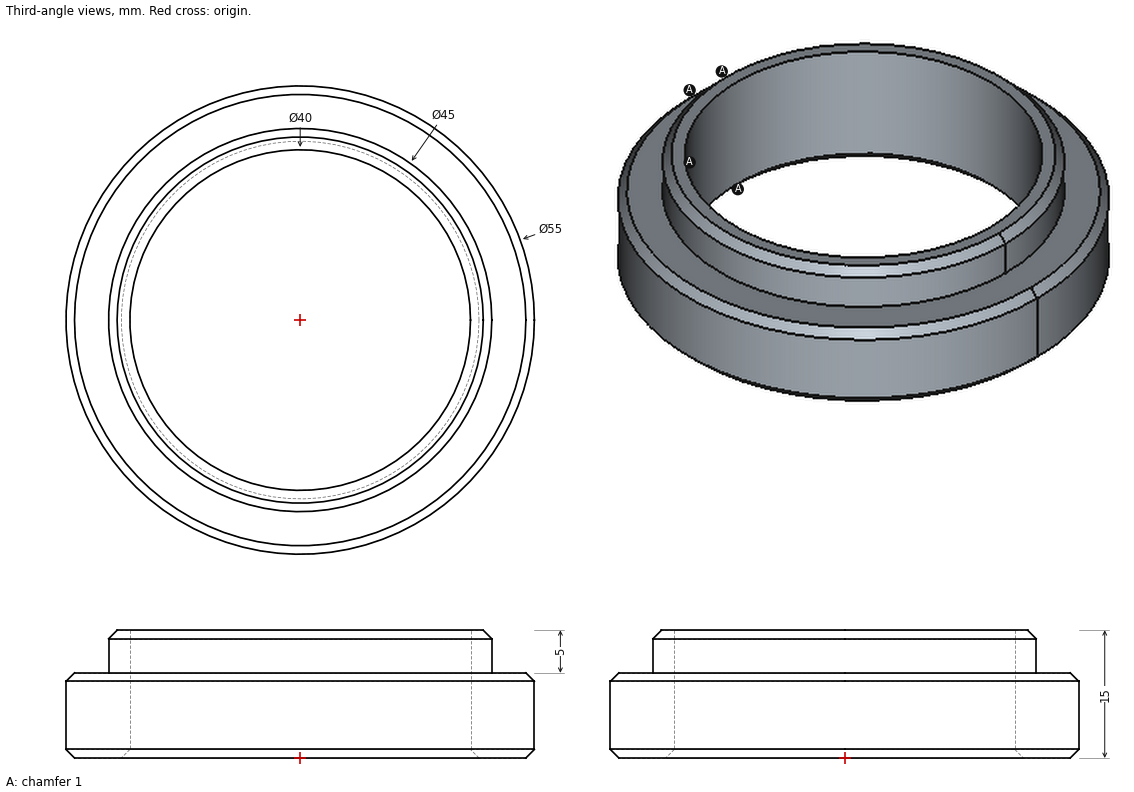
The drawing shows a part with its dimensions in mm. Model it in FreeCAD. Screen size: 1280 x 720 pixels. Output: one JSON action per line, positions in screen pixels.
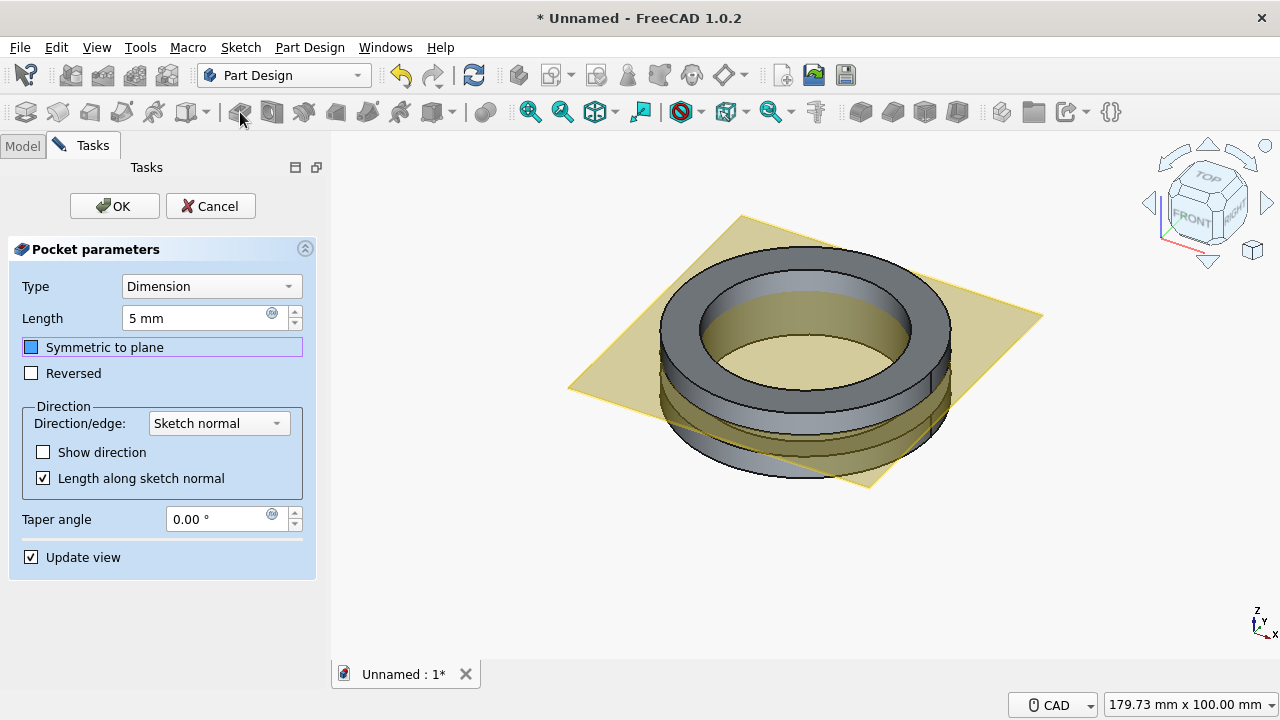
{"action": "left_click", "coordinate": [30, 373]}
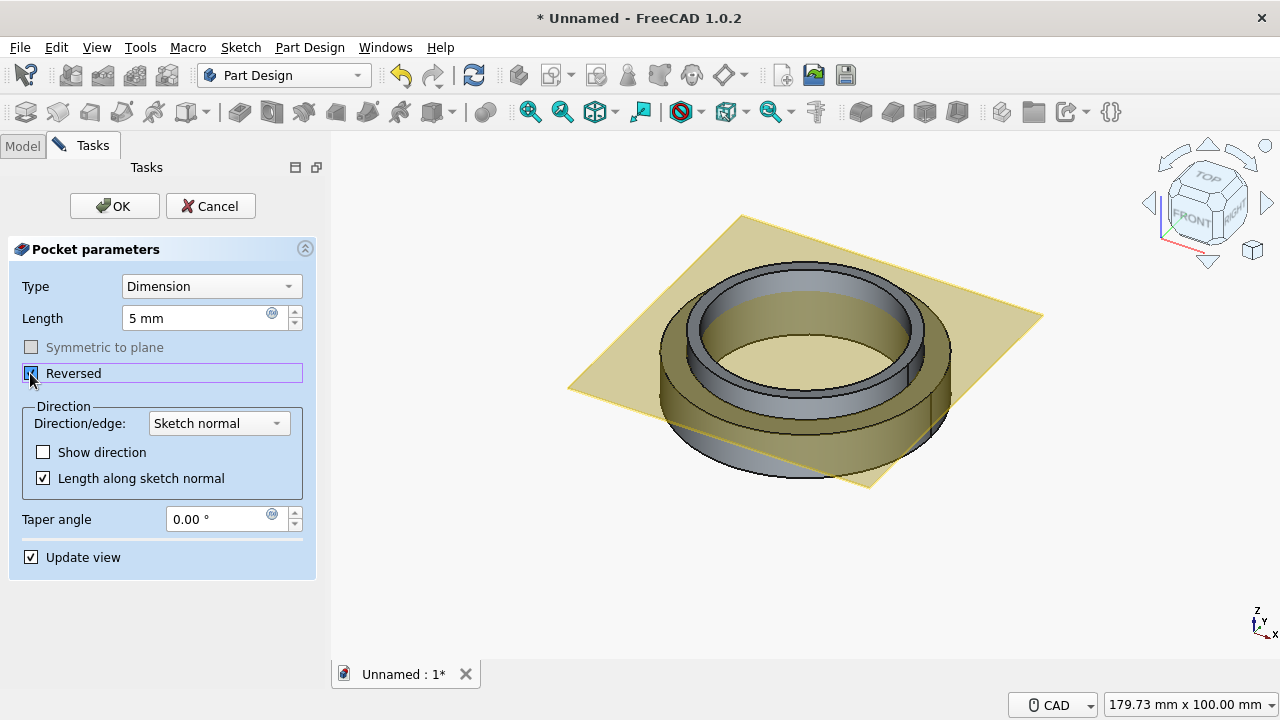
{"action": "left_click", "coordinate": [115, 206]}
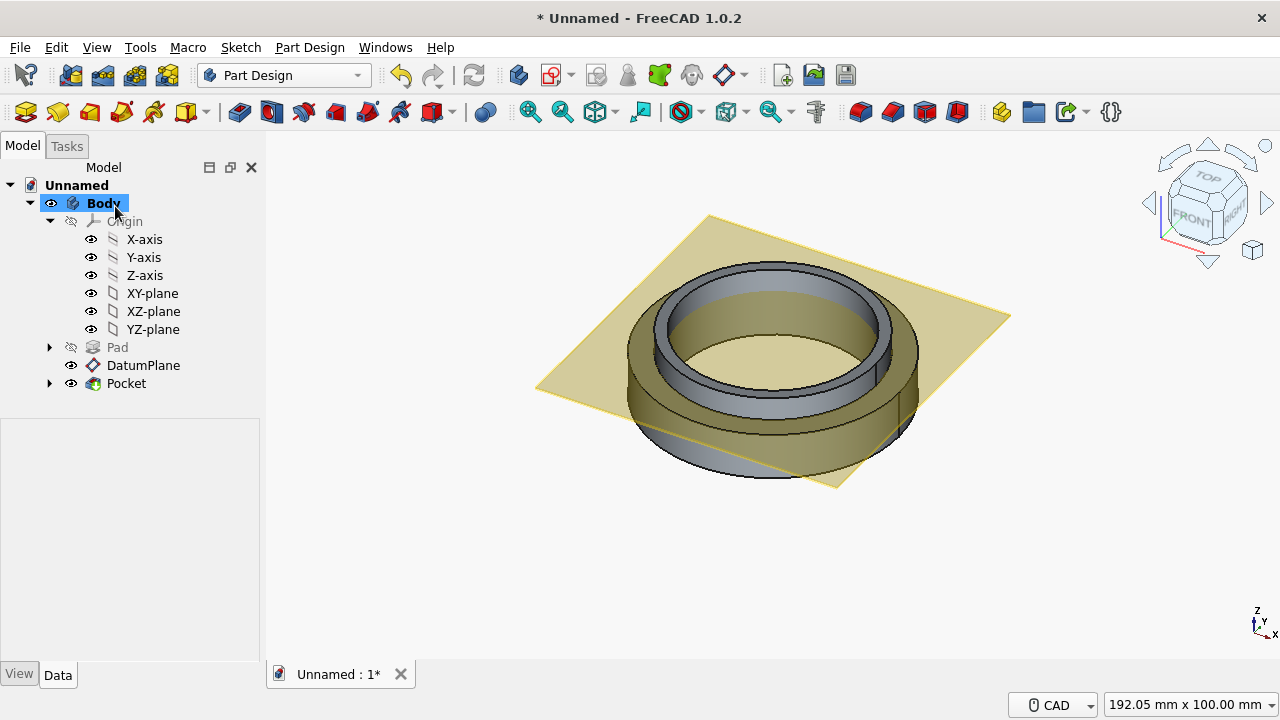
{"action": "left_click", "coordinate": [116, 365]}
{"action": "key", "text": "space"}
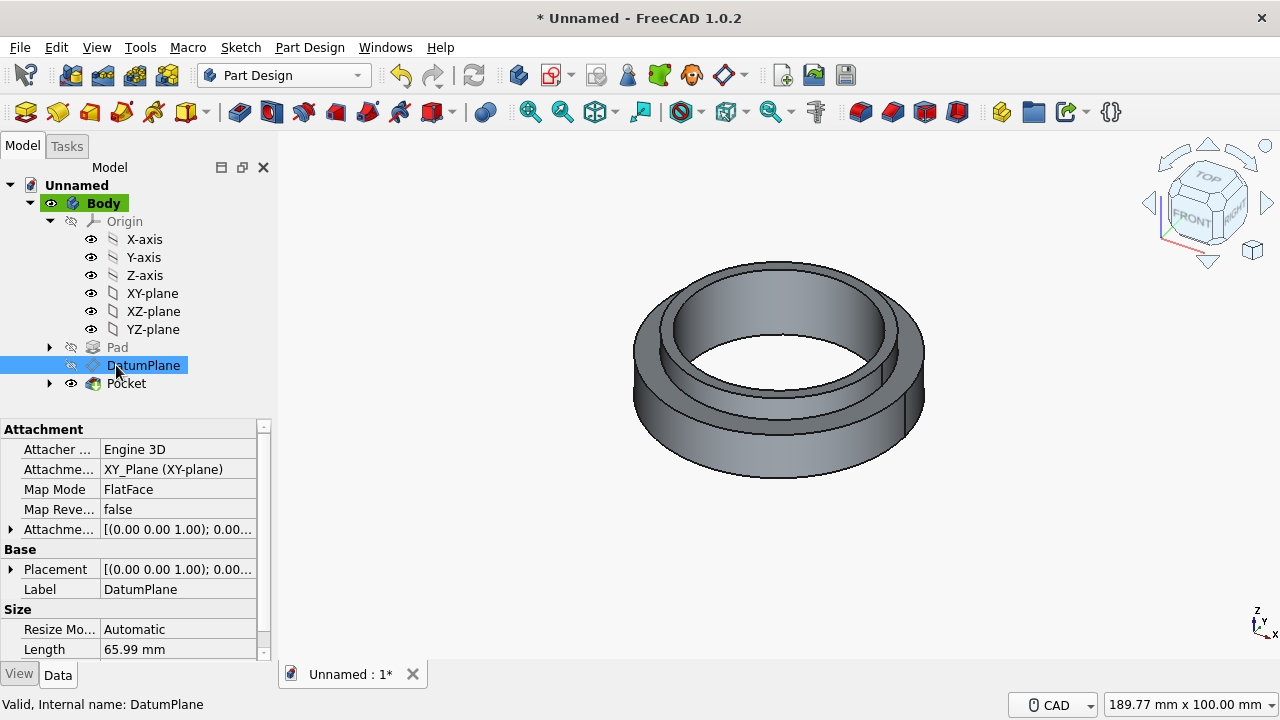
{"action": "left_click", "coordinate": [635, 359]}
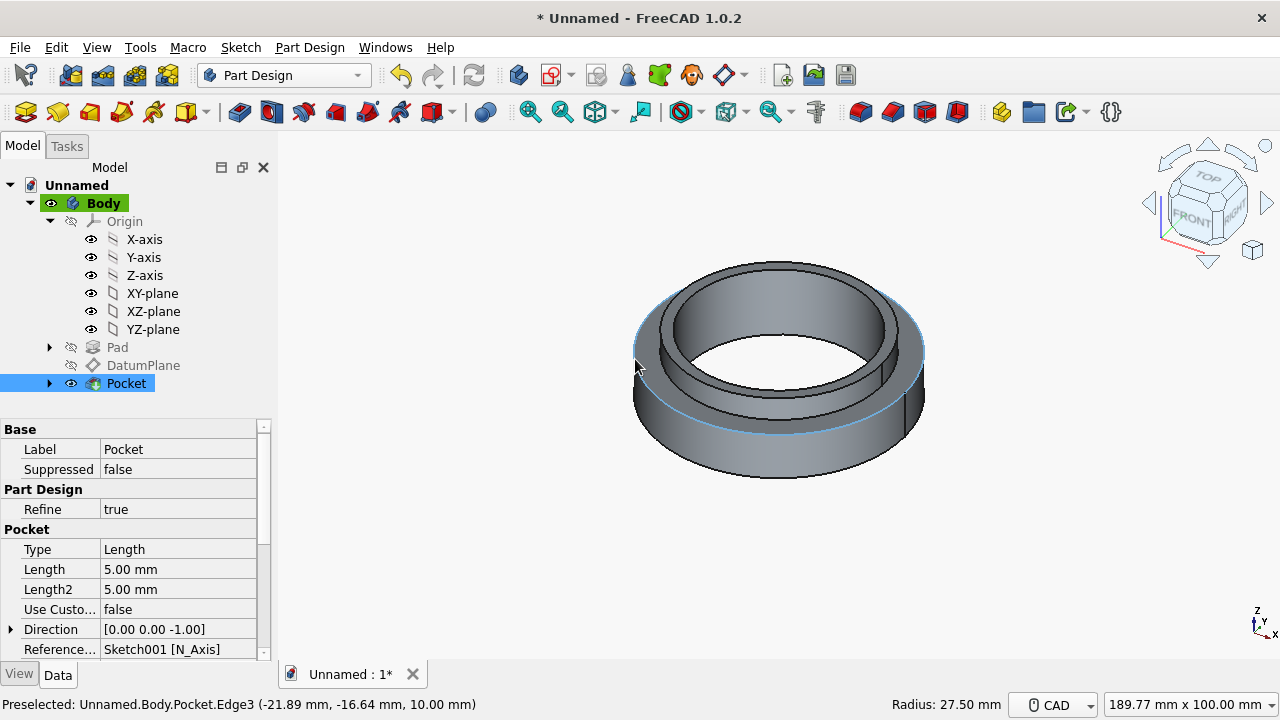
{"action": "left_click", "coordinate": [661, 336], "text": "ctrl"}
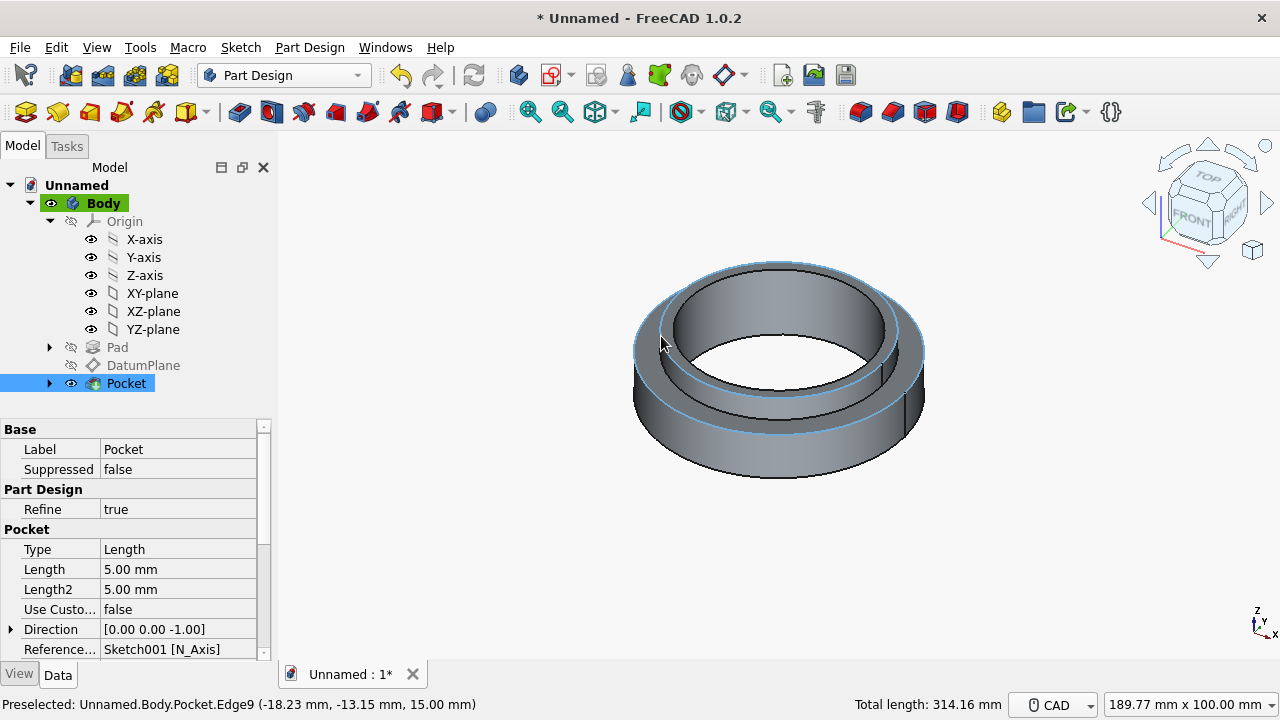
{"action": "key", "text": "0"}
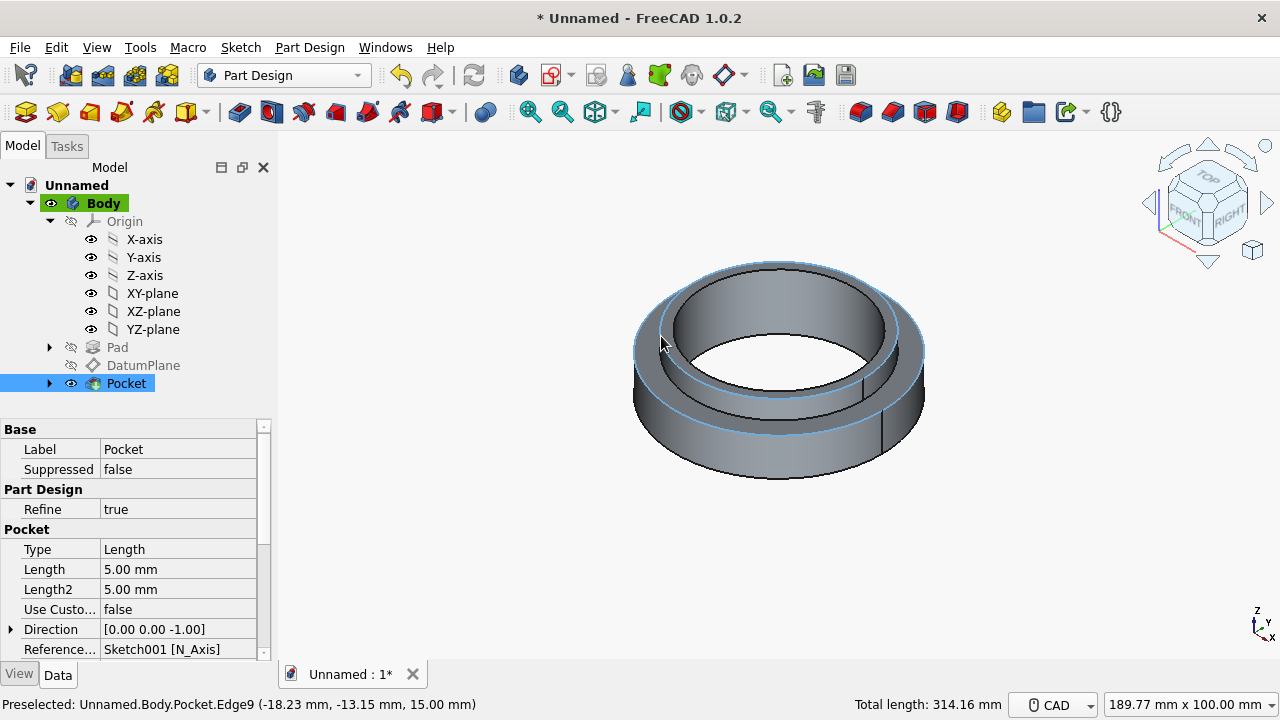
{"action": "key", "text": "2"}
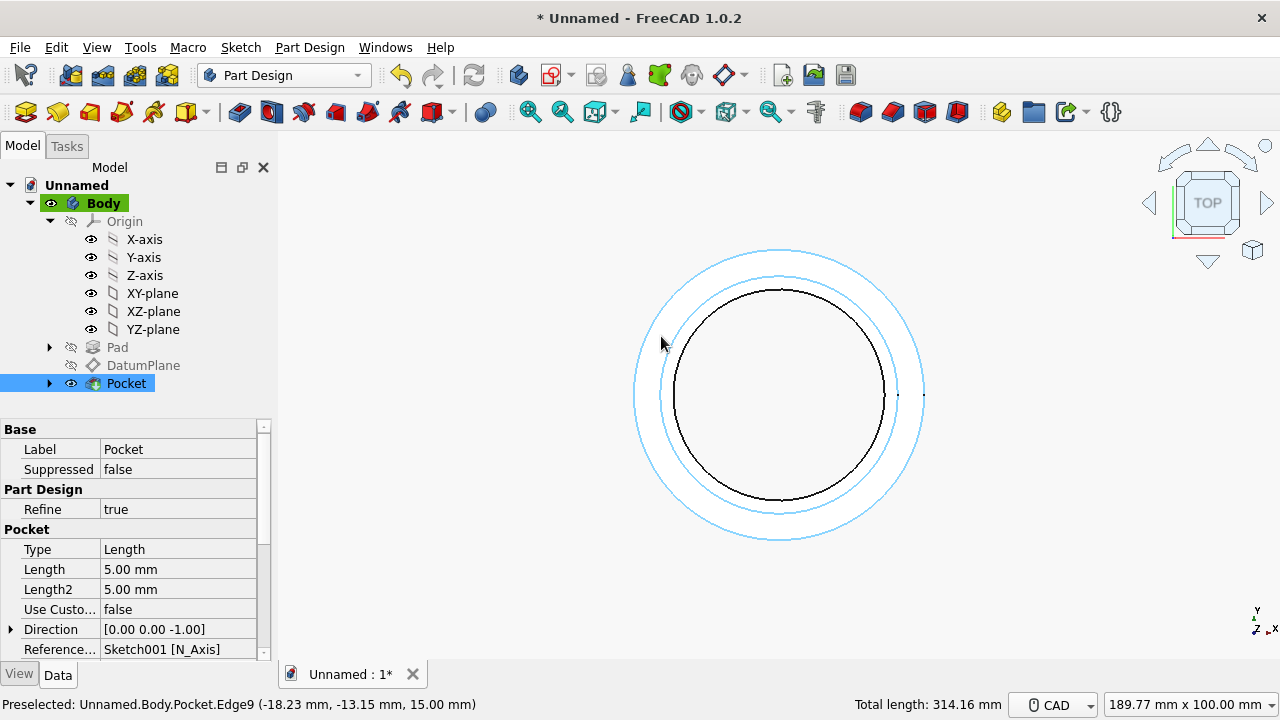
{"action": "key", "text": "1"}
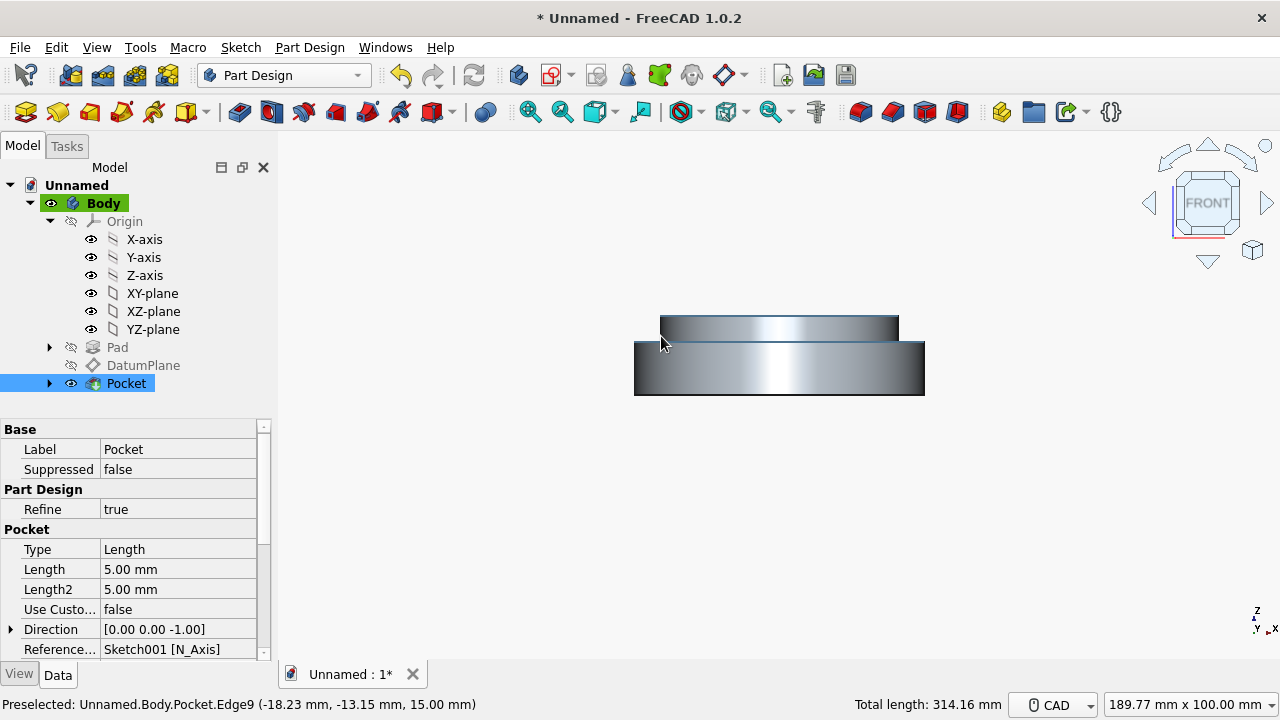
{"action": "key", "text": "v f"}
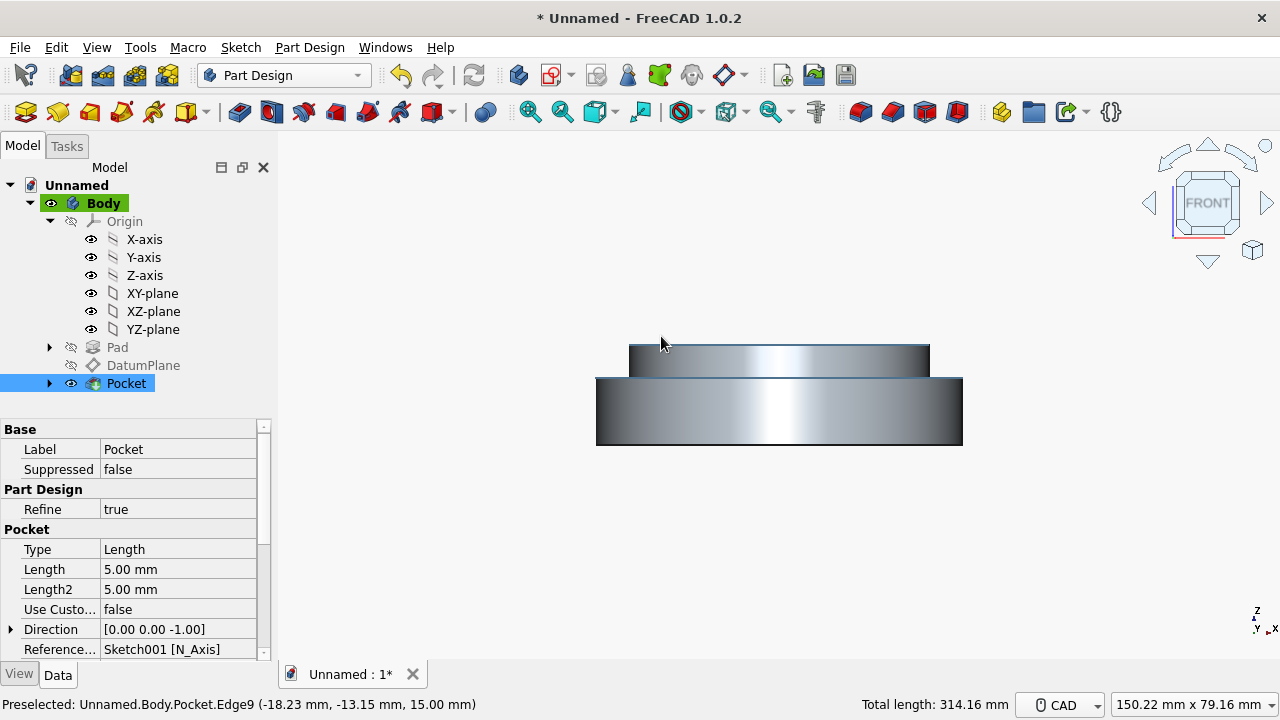
{"action": "left_click", "coordinate": [631, 444], "text": "ctrl"}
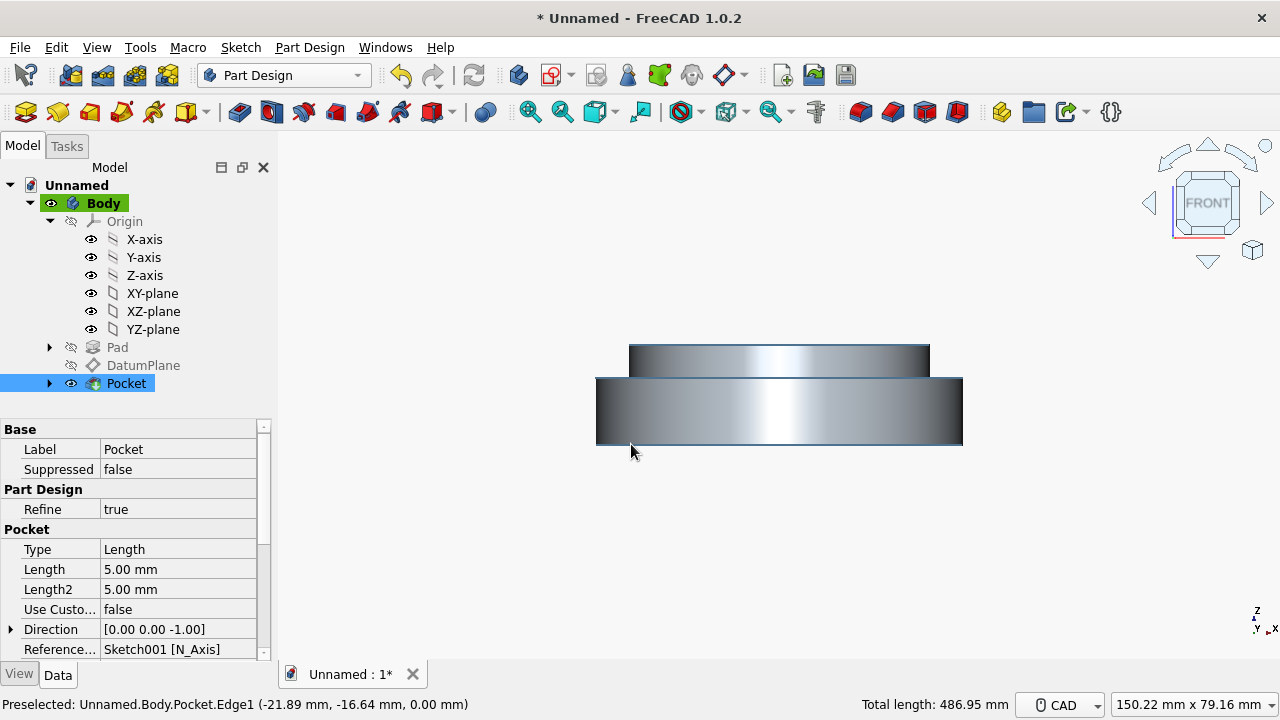
{"action": "key", "text": "3"}